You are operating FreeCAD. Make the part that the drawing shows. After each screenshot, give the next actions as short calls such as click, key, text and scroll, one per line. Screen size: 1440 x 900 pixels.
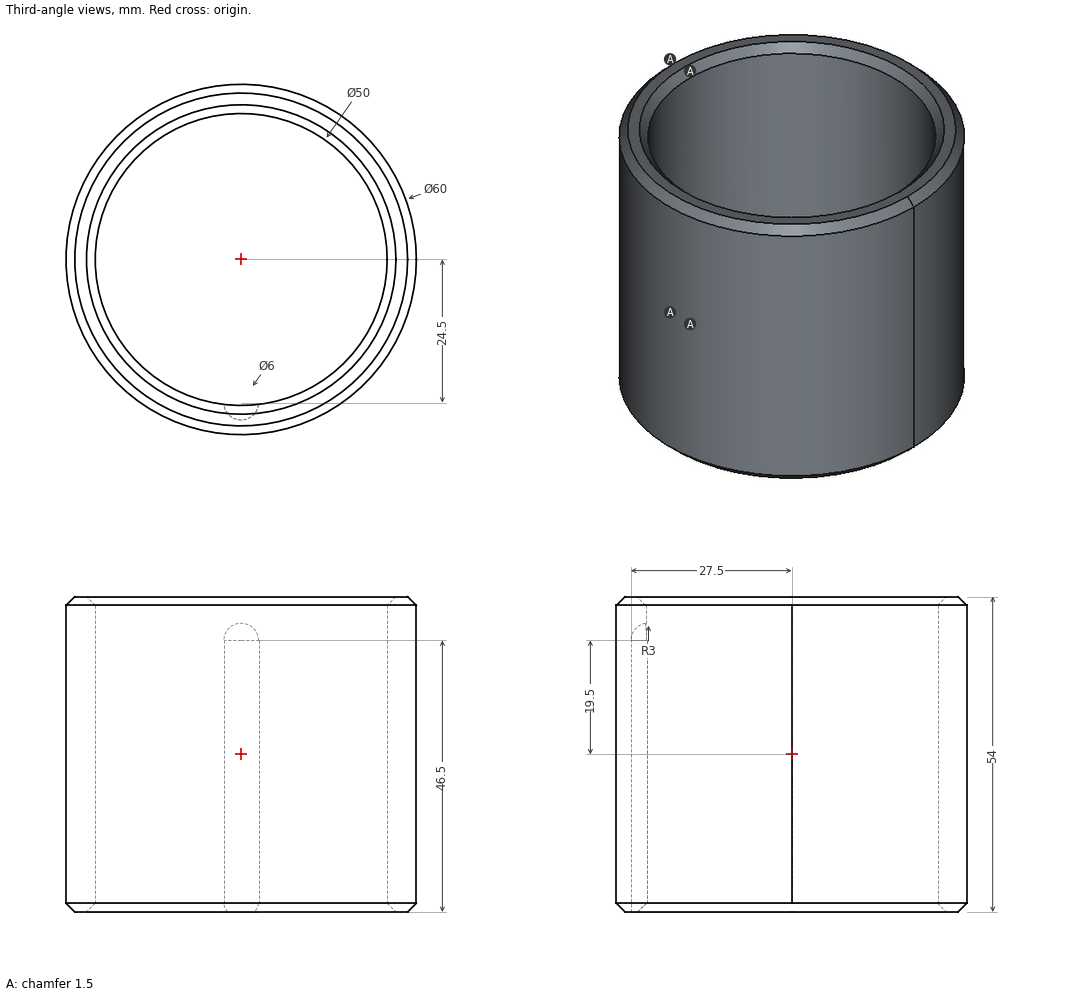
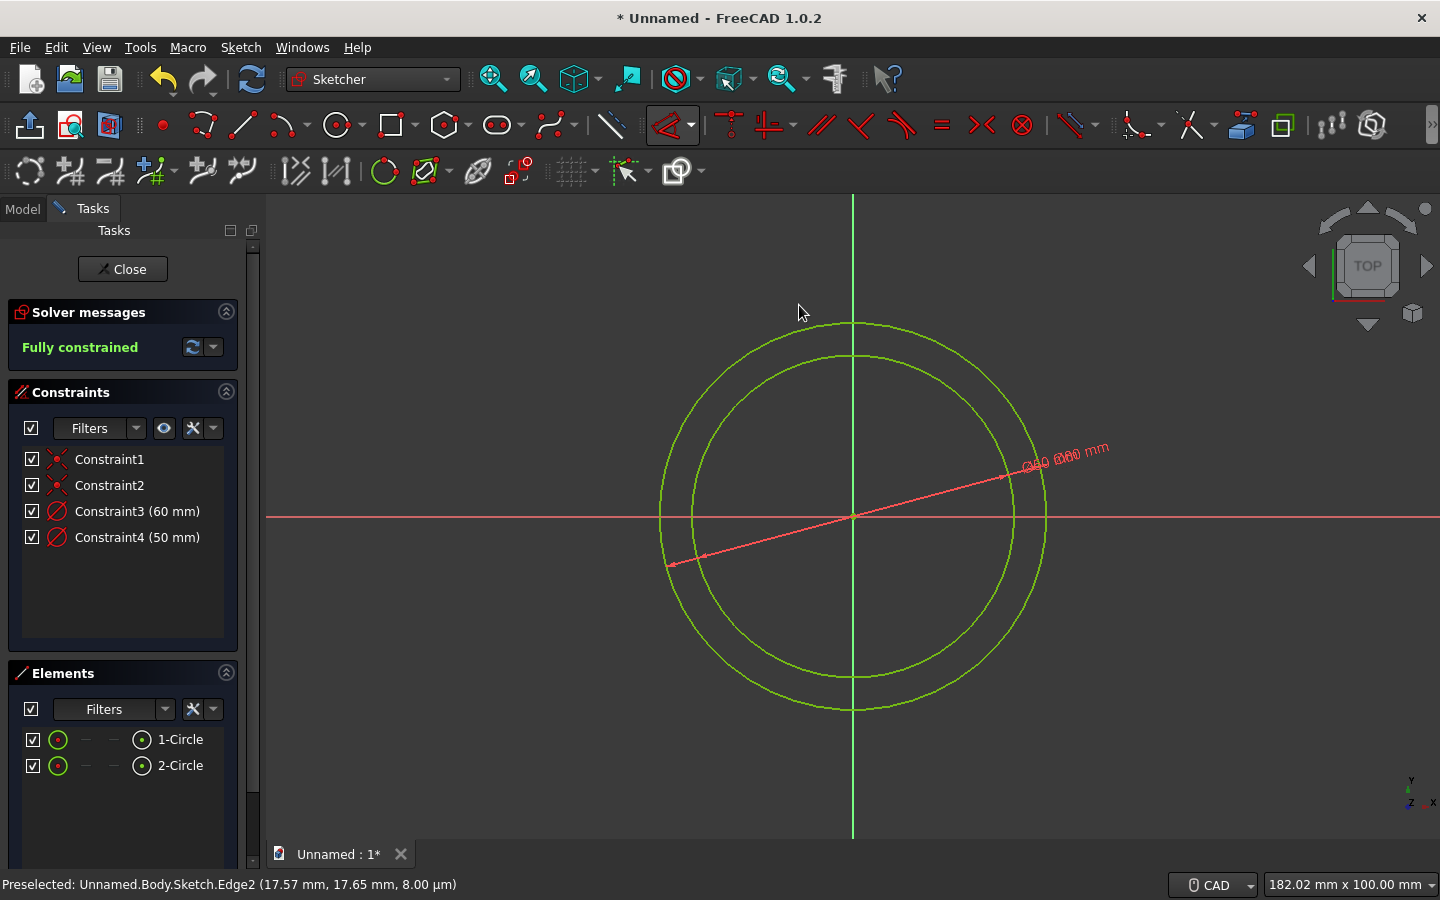
click(123, 269)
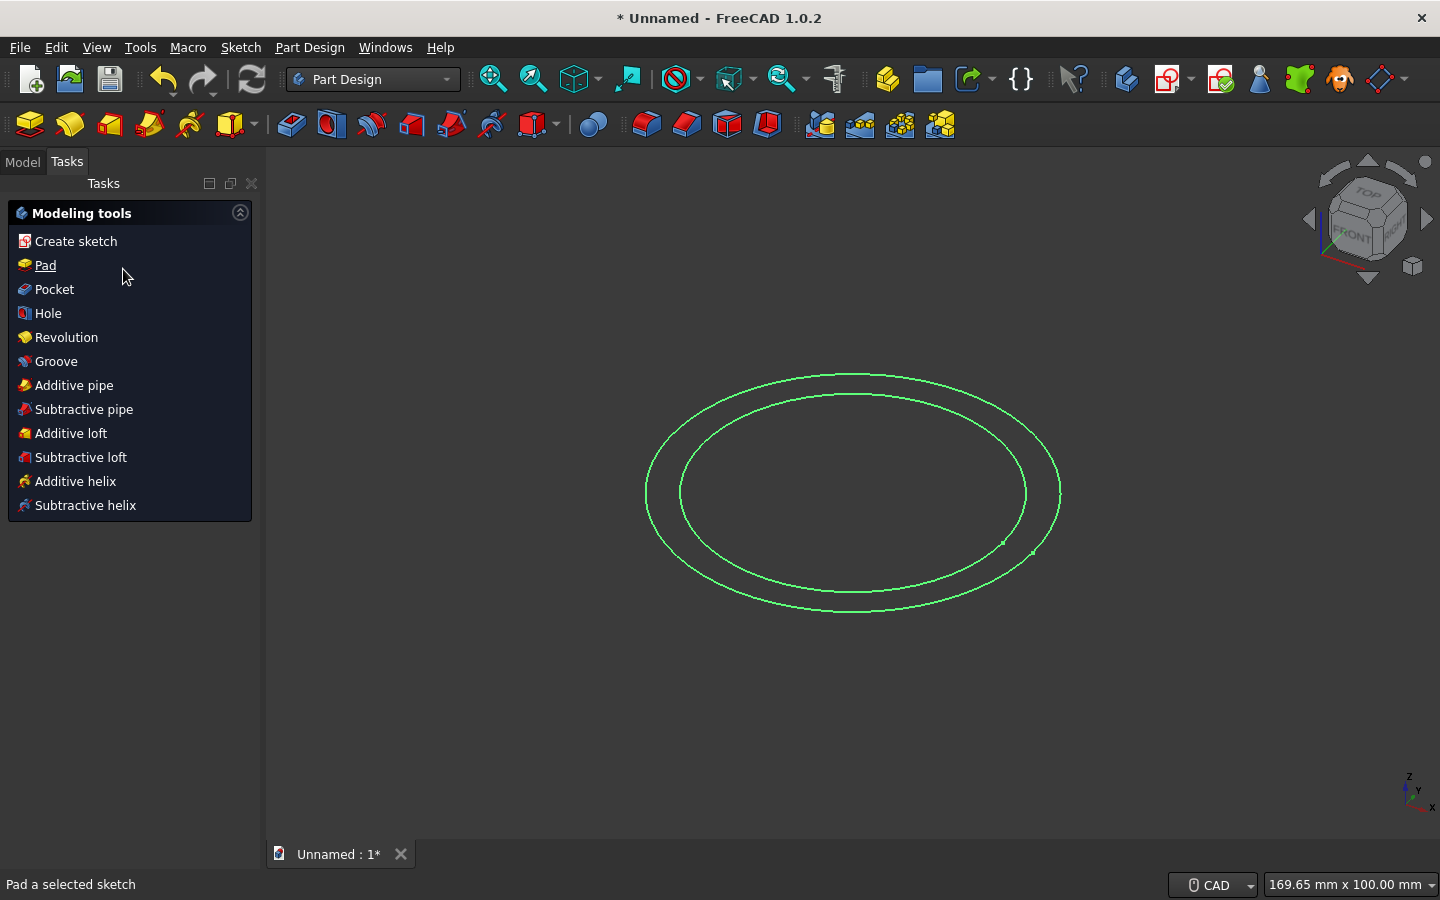
click(30, 124)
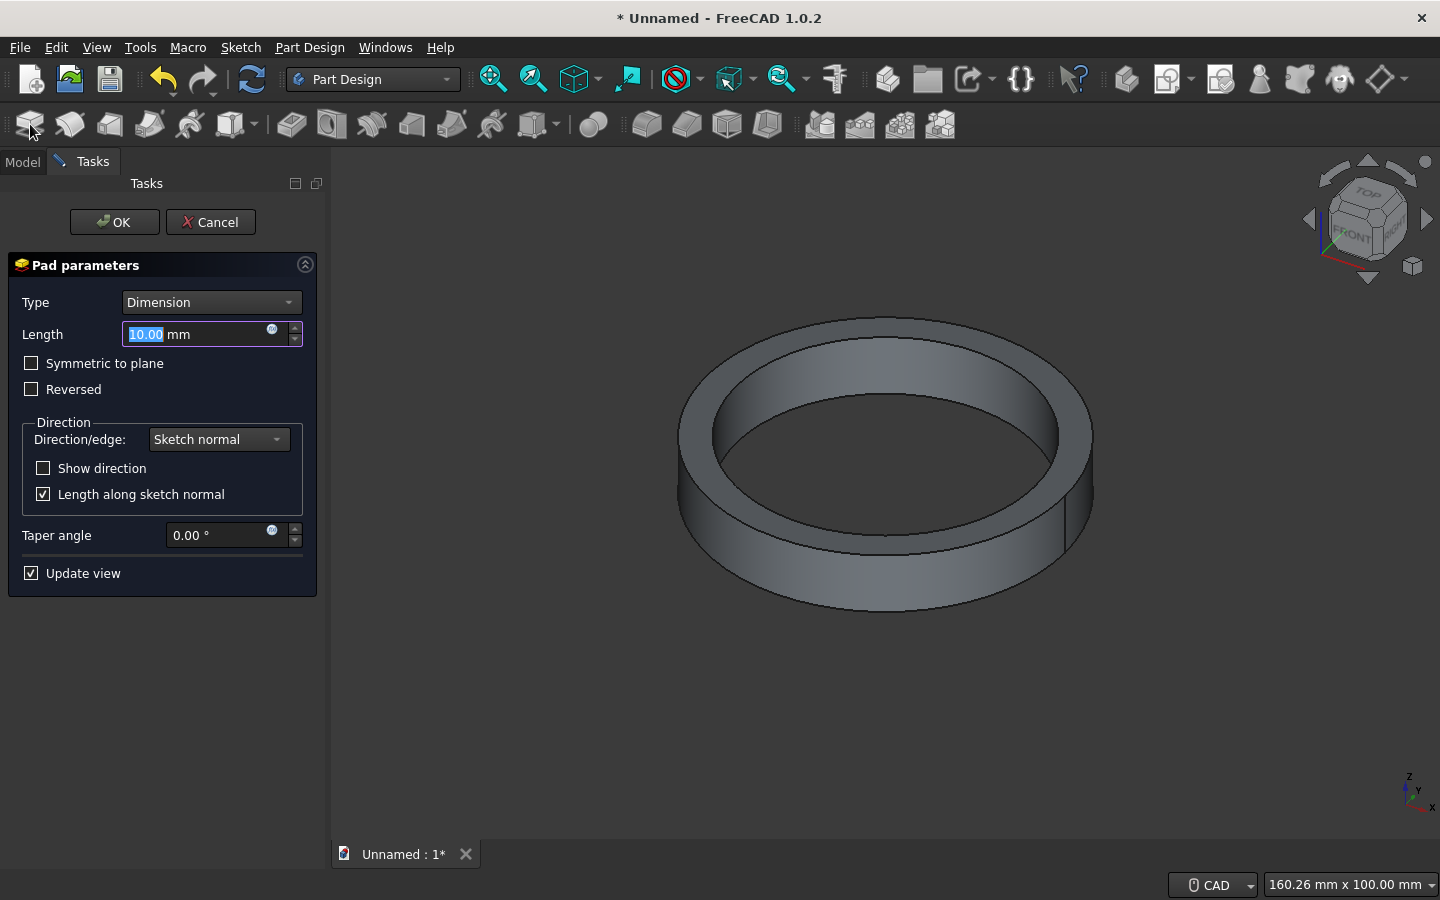
text(54)
key(Tab)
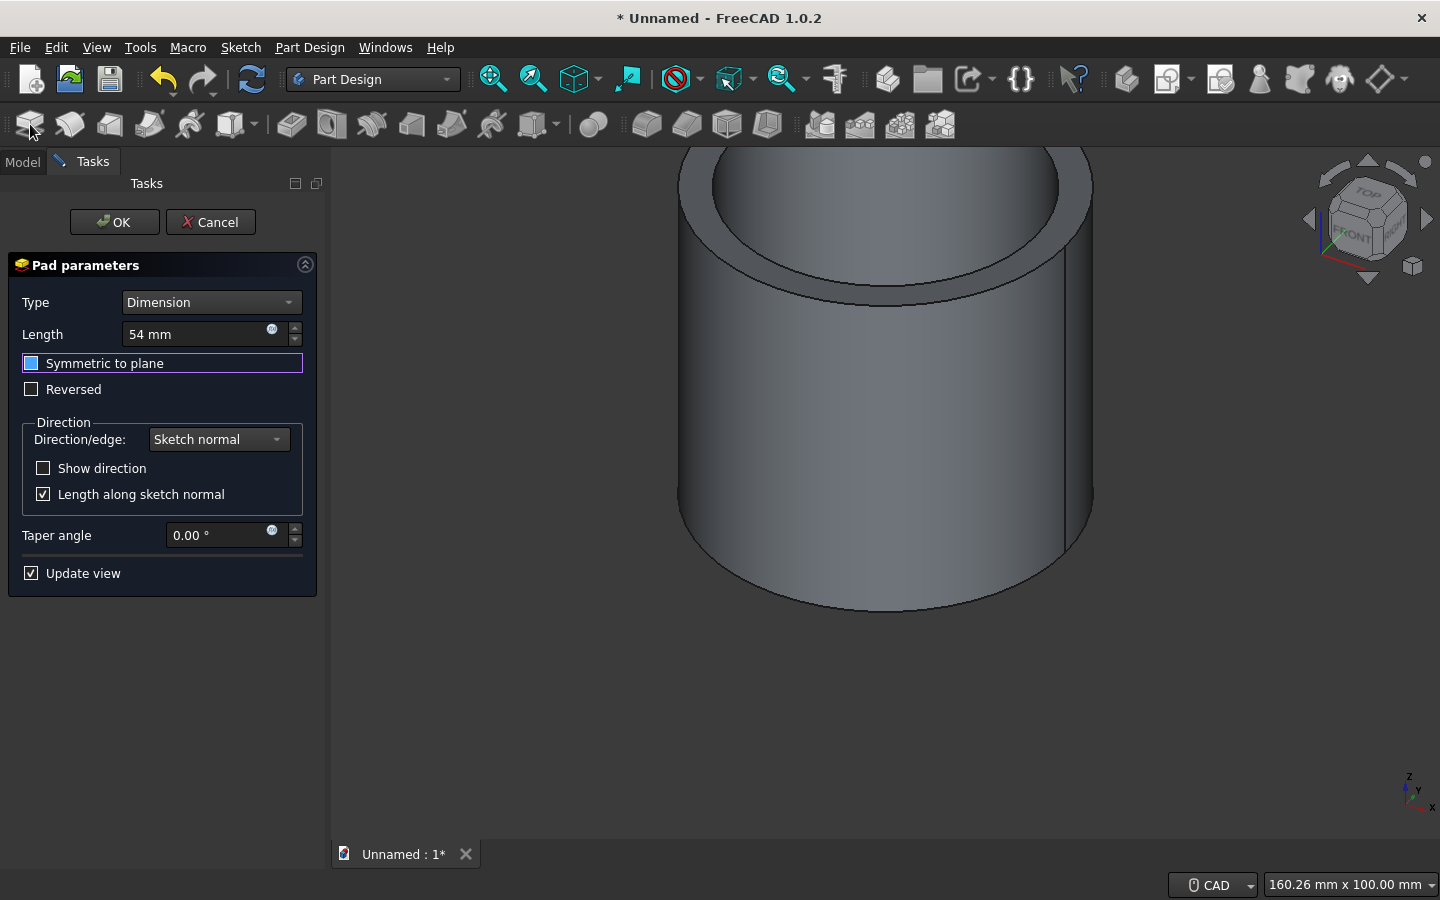
click(30, 363)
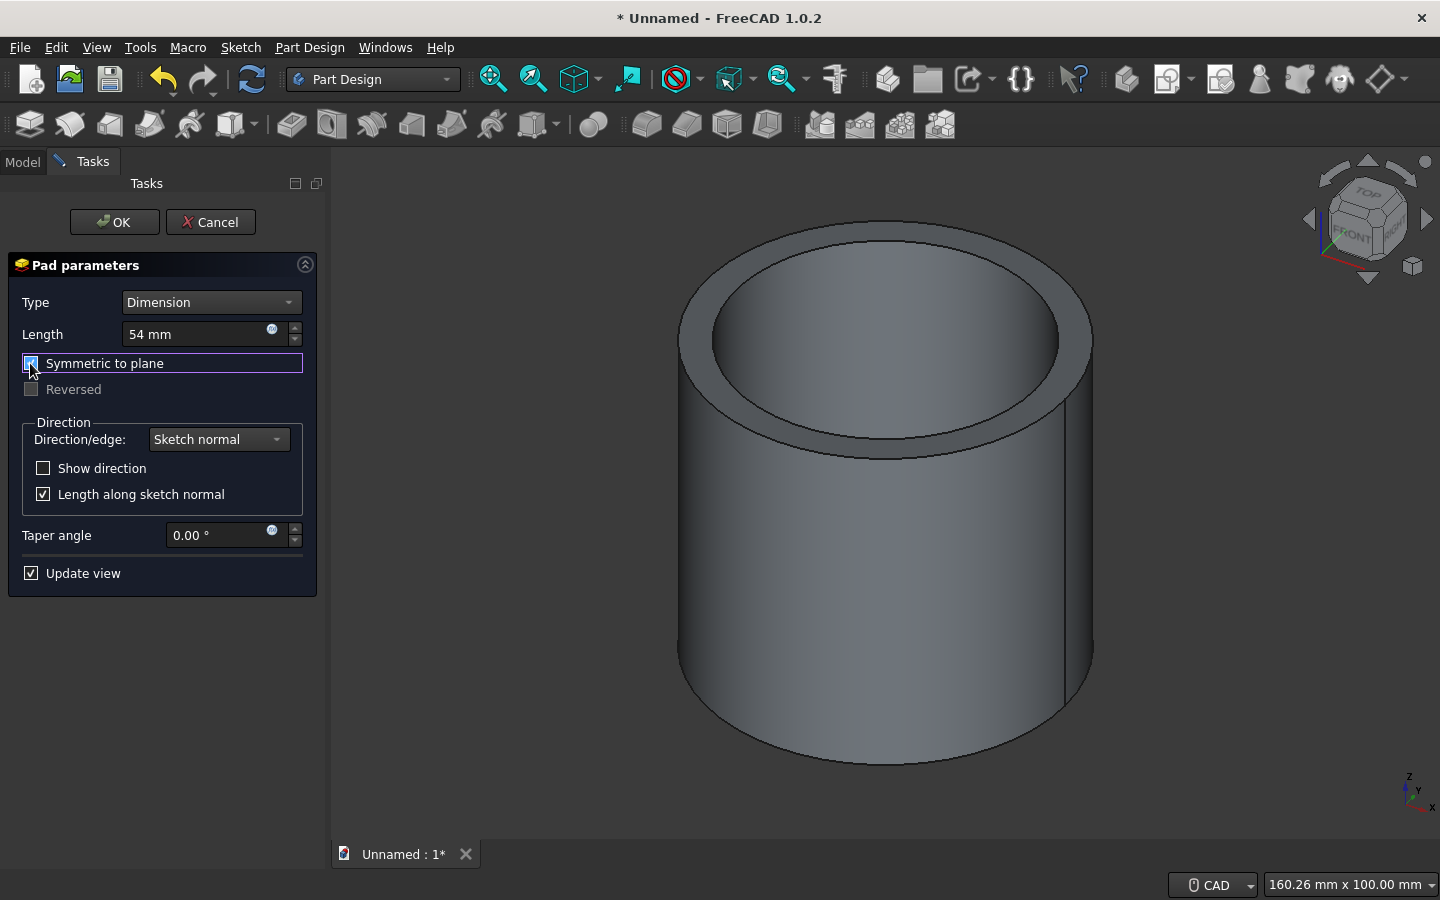
click(115, 222)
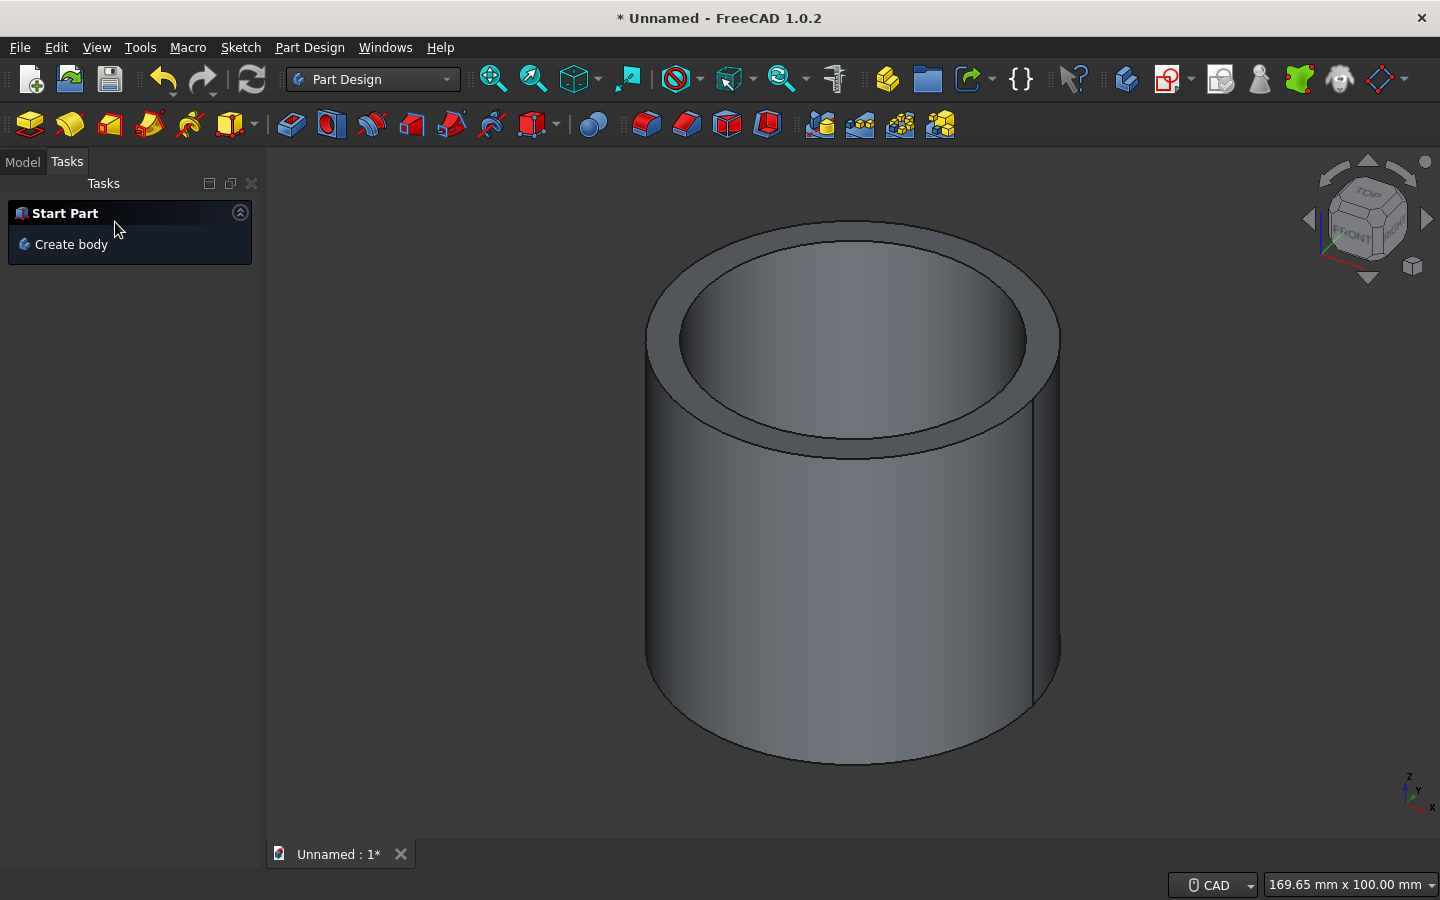
click(647, 351)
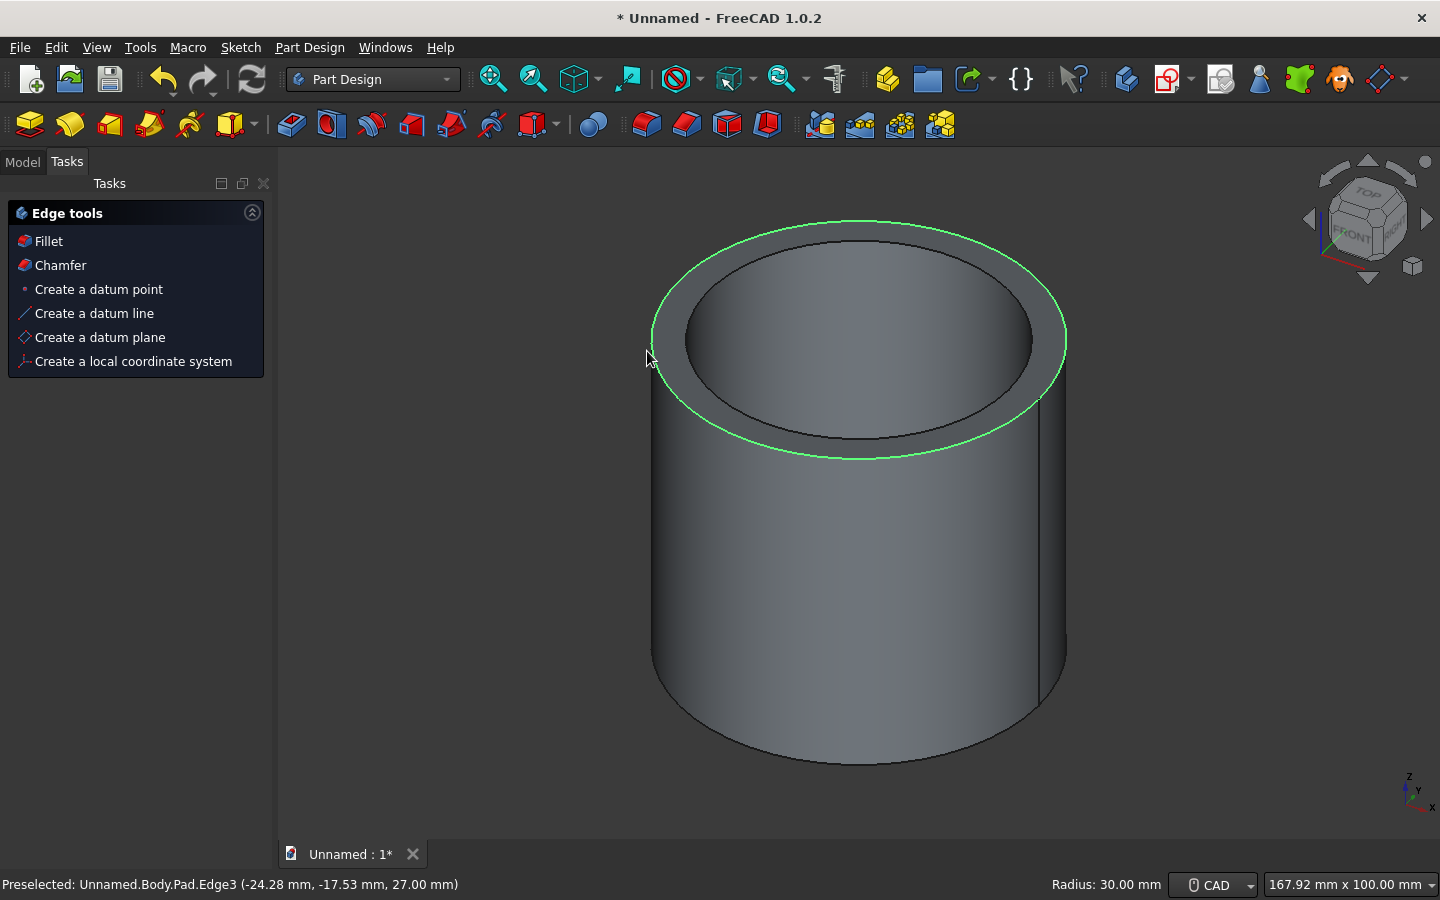
click(709, 289, ctrl)